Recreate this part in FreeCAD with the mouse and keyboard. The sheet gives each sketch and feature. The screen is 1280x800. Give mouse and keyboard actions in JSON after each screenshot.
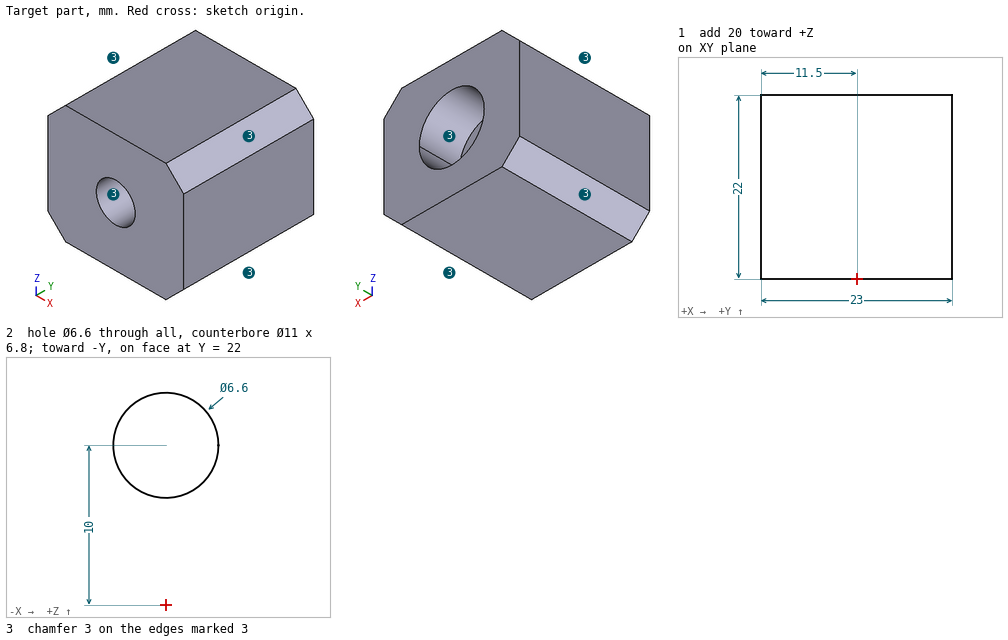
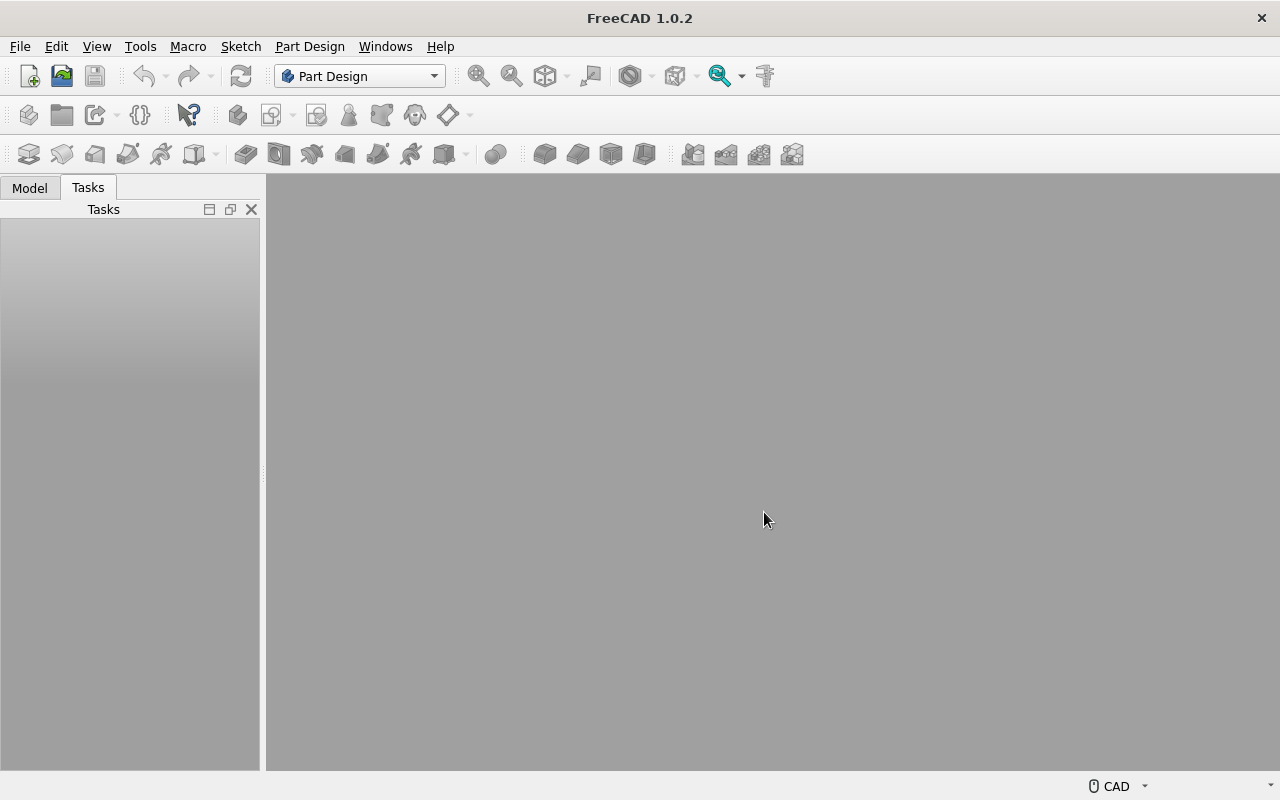
{"action": "left_click", "coordinate": [29, 76]}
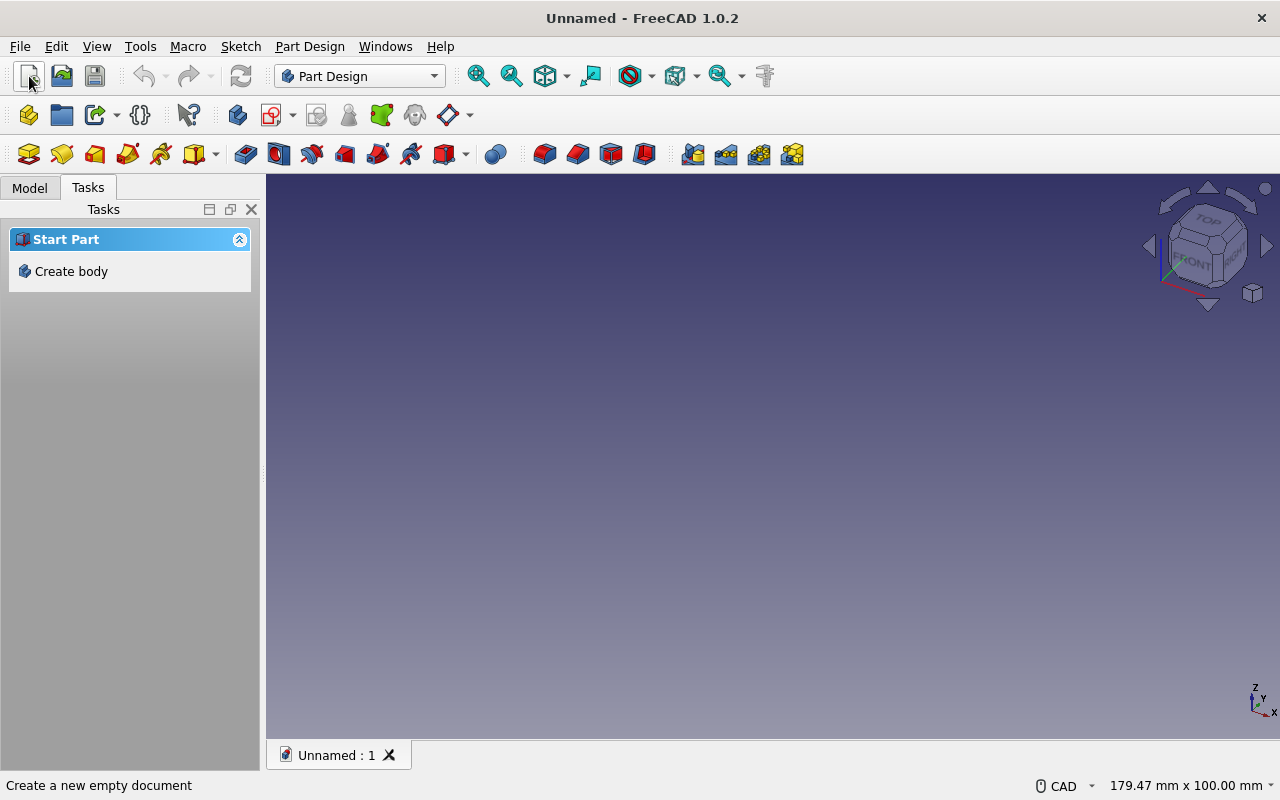
{"action": "left_click", "coordinate": [270, 116]}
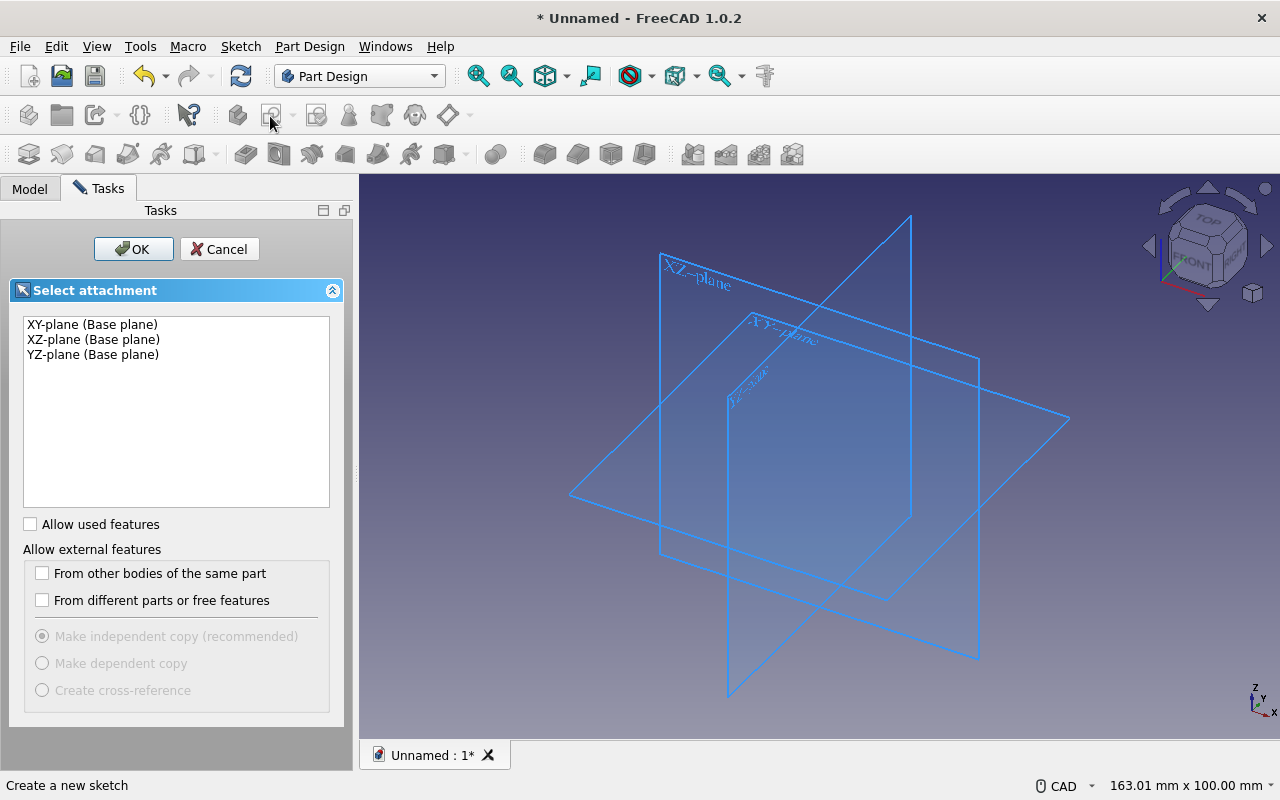
{"action": "left_click", "coordinate": [84, 324]}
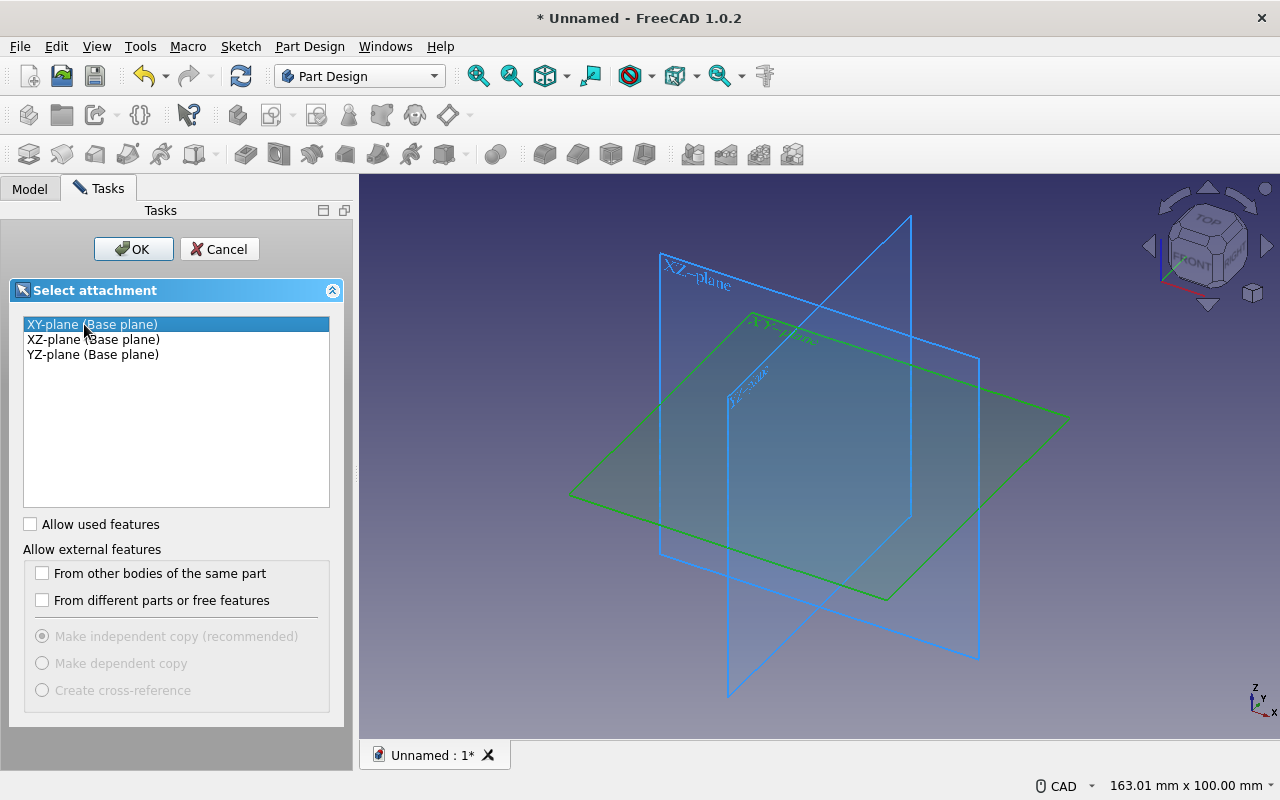
{"action": "left_click", "coordinate": [134, 249]}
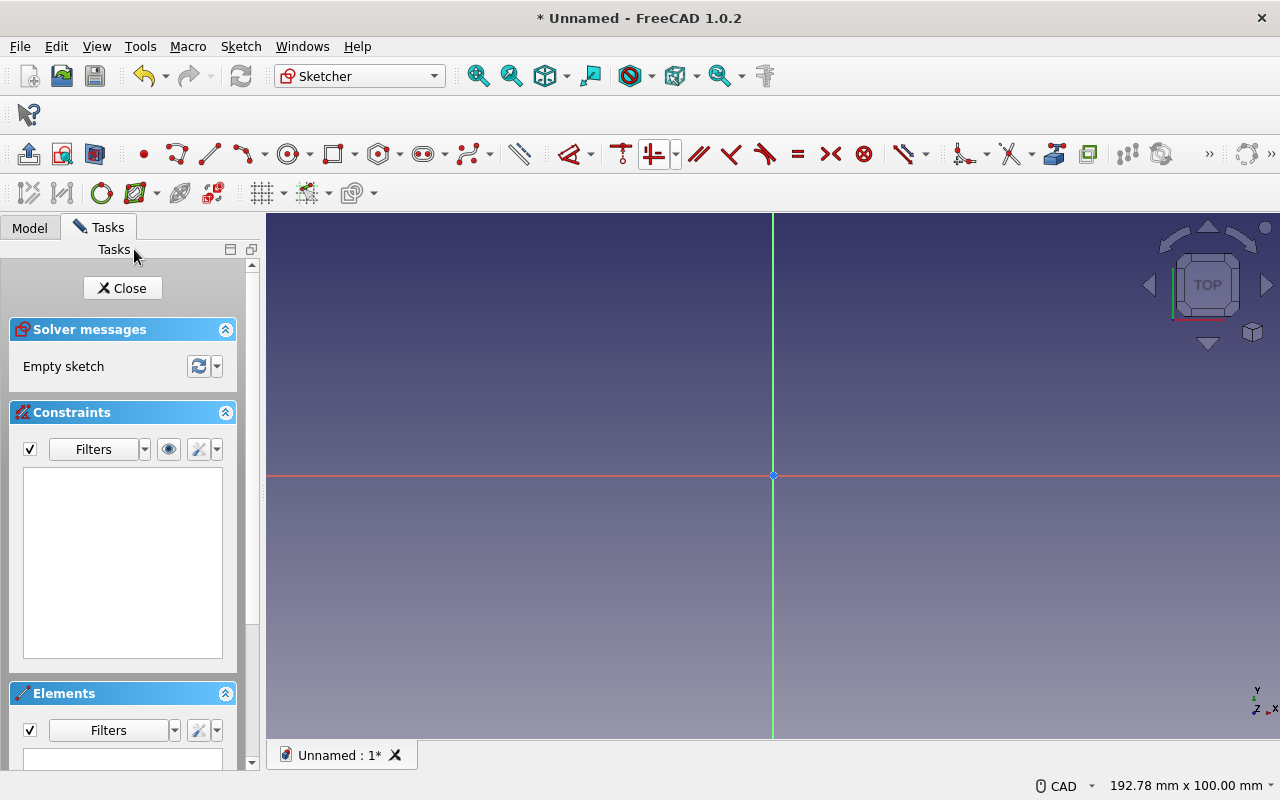
{"action": "scroll", "coordinate": [813, 384], "scroll_direction": "up", "scroll_amount": 5}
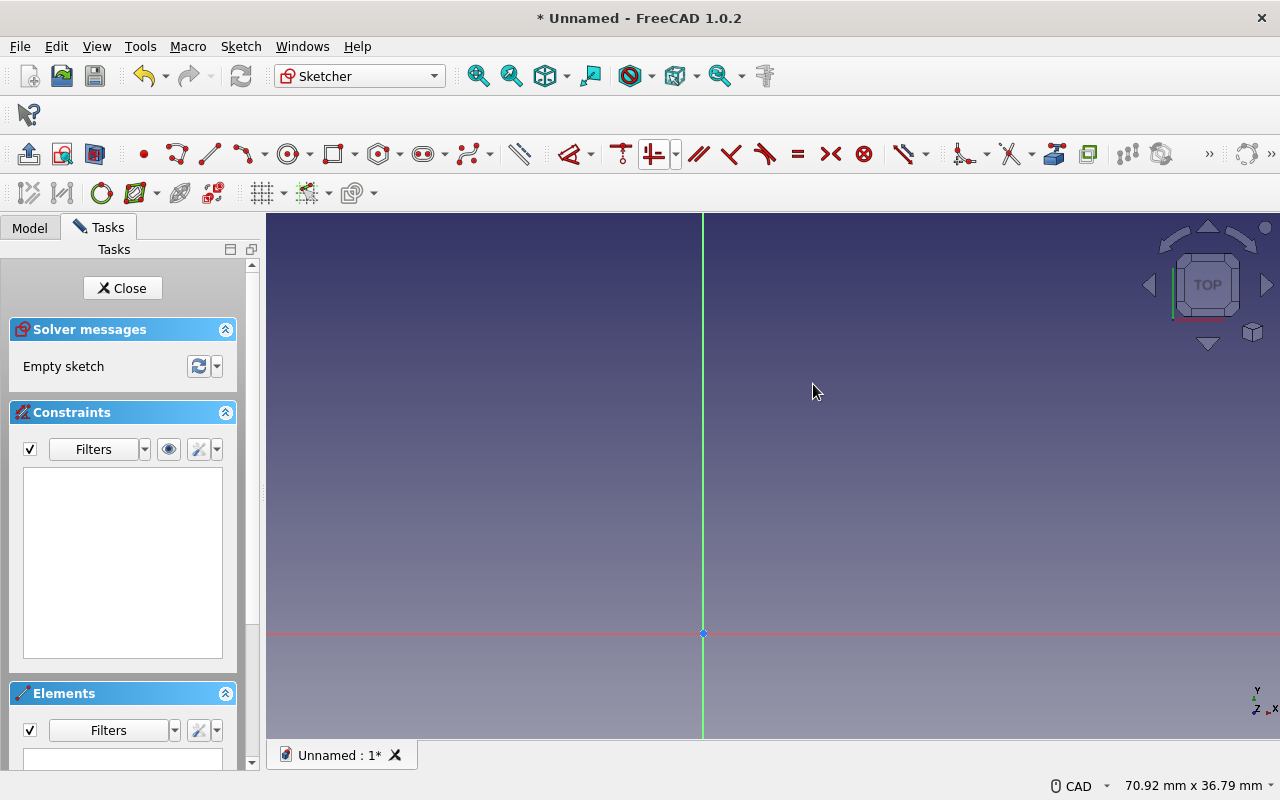
{"action": "left_click", "coordinate": [332, 154]}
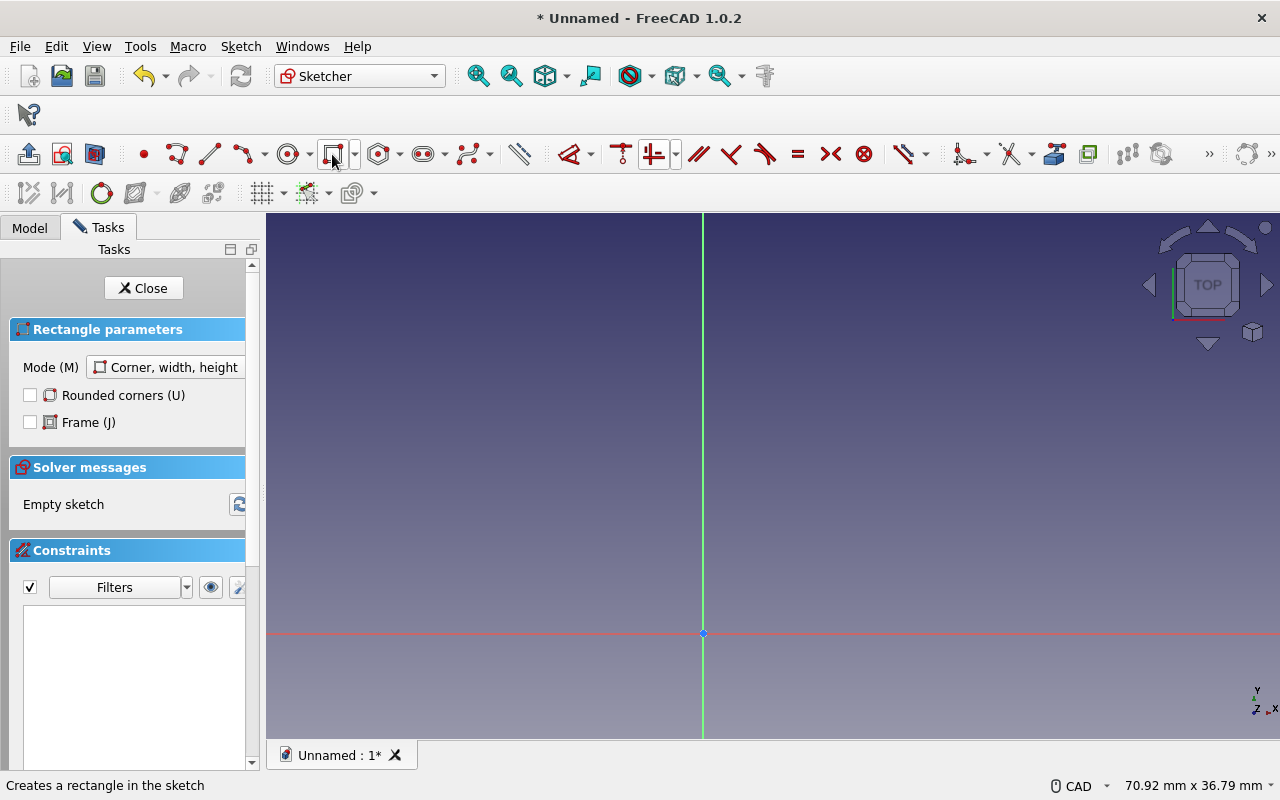
{"action": "left_click", "coordinate": [539, 319]}
{"action": "left_click", "coordinate": [868, 634]}
{"action": "key", "text": "Escape"}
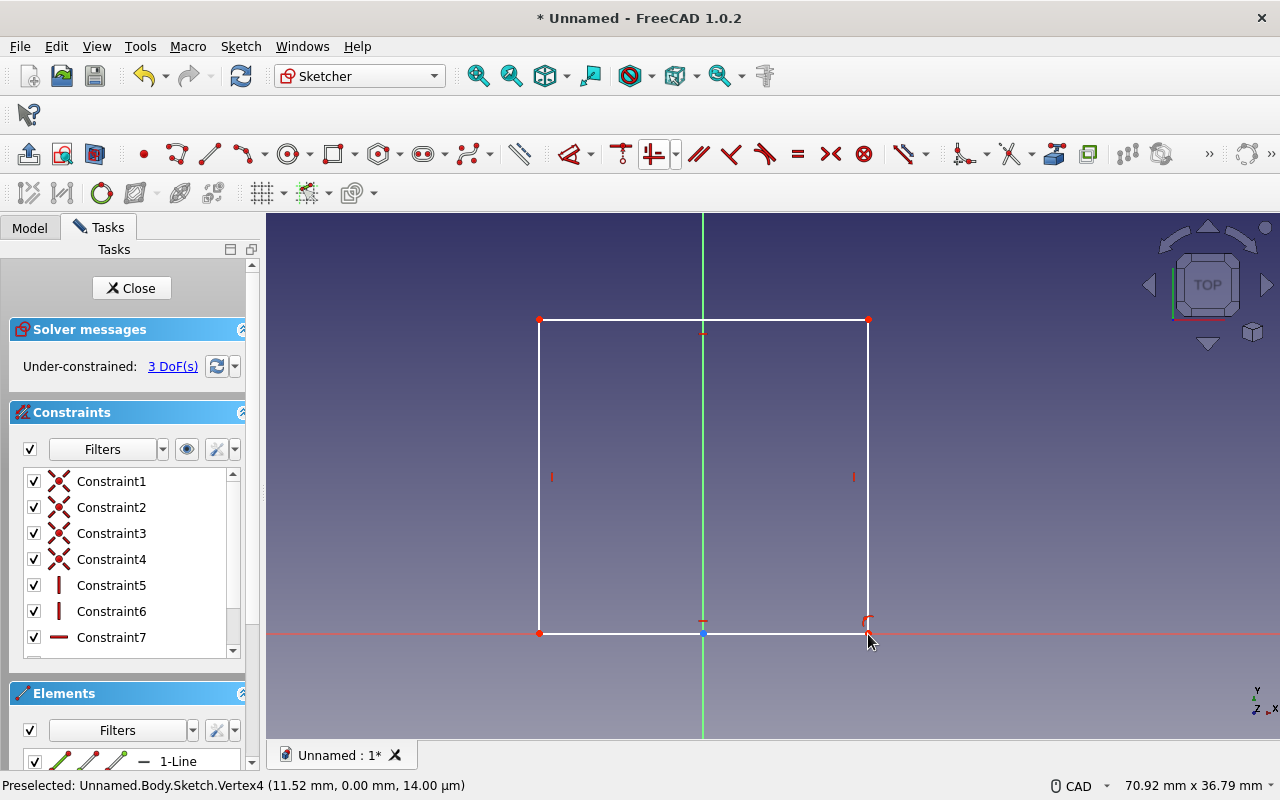
{"action": "left_click", "coordinate": [568, 154]}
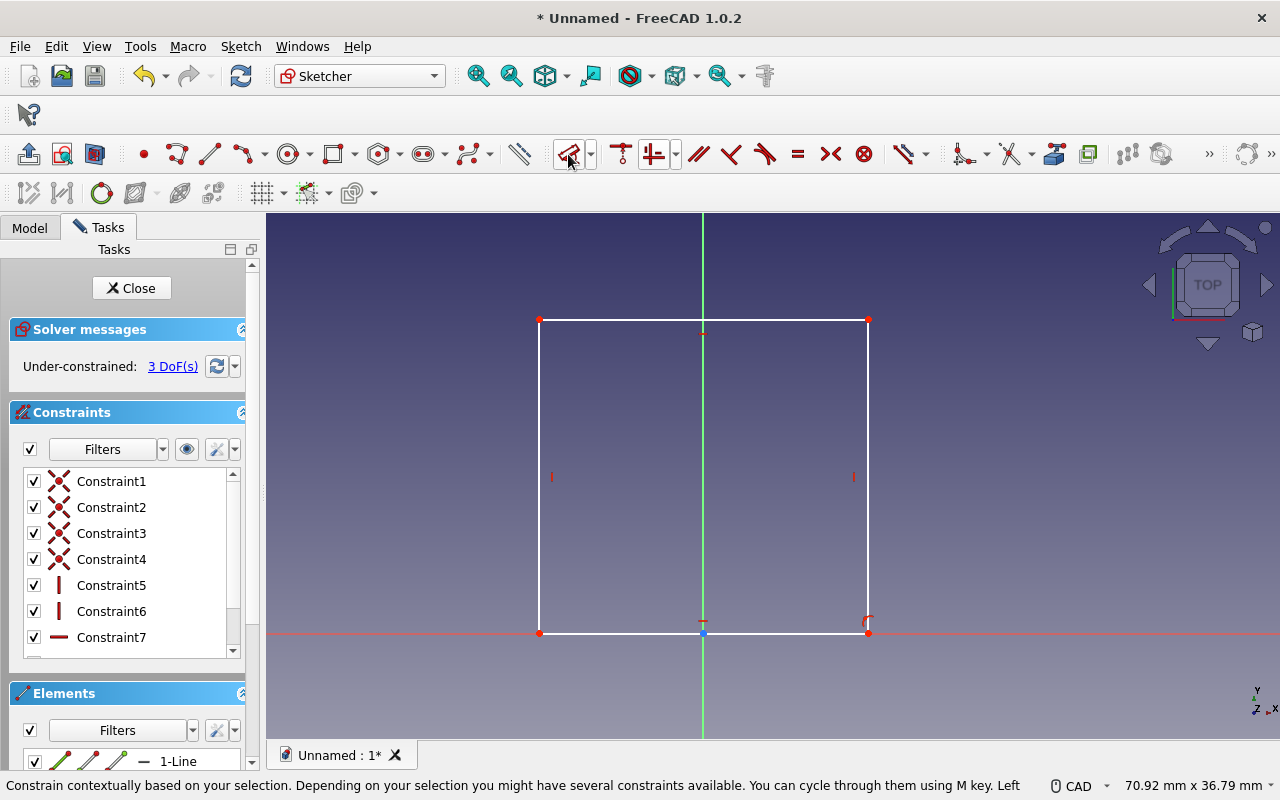
{"action": "left_click", "coordinate": [539, 414]}
{"action": "left_click", "coordinate": [505, 477]}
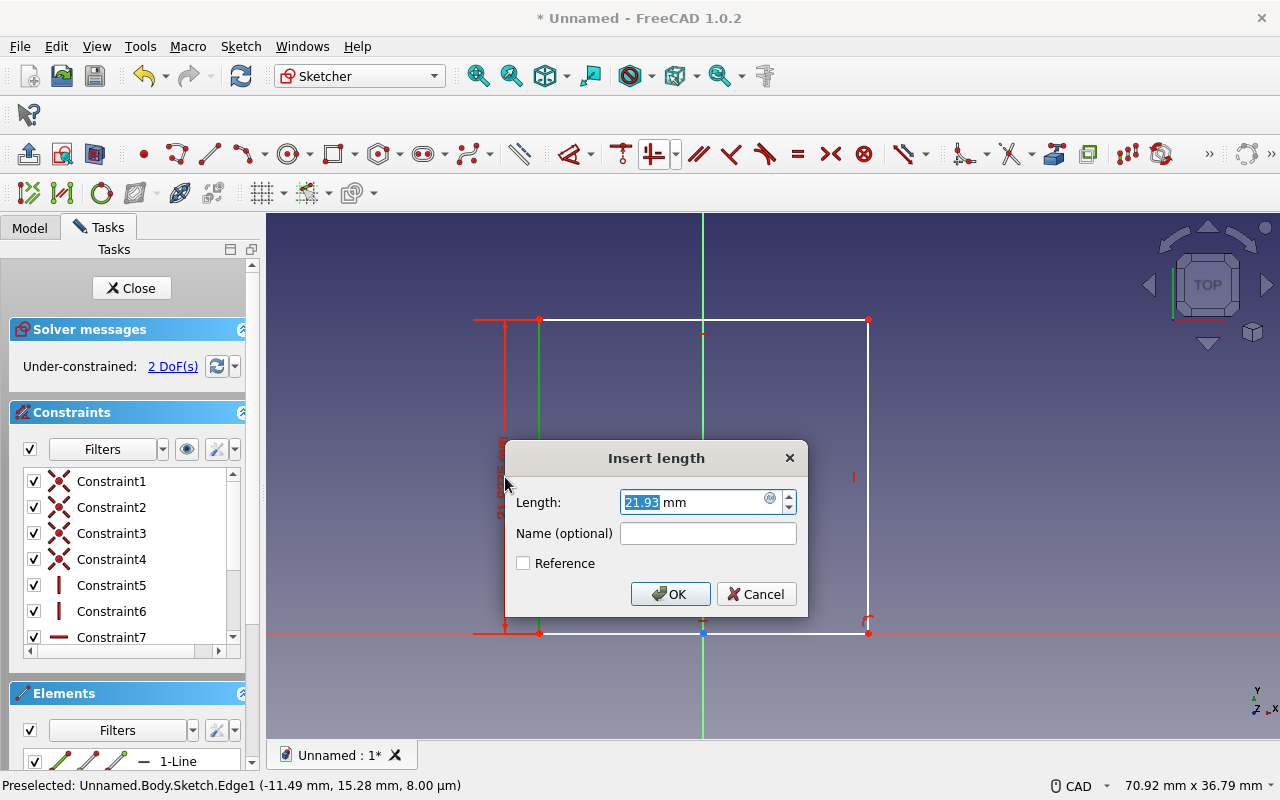
{"action": "type", "text": "22"}
{"action": "key", "text": "Return"}